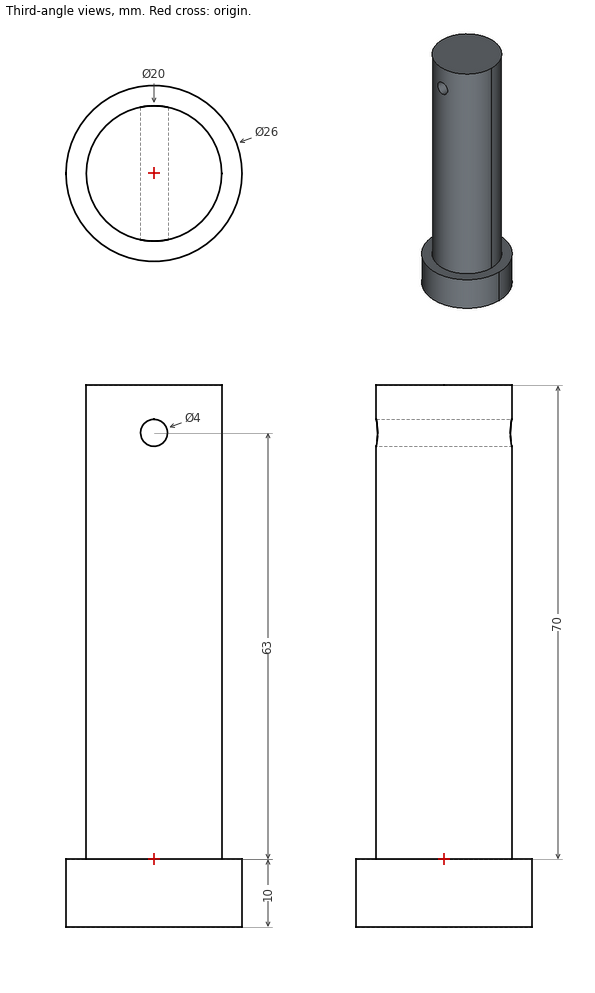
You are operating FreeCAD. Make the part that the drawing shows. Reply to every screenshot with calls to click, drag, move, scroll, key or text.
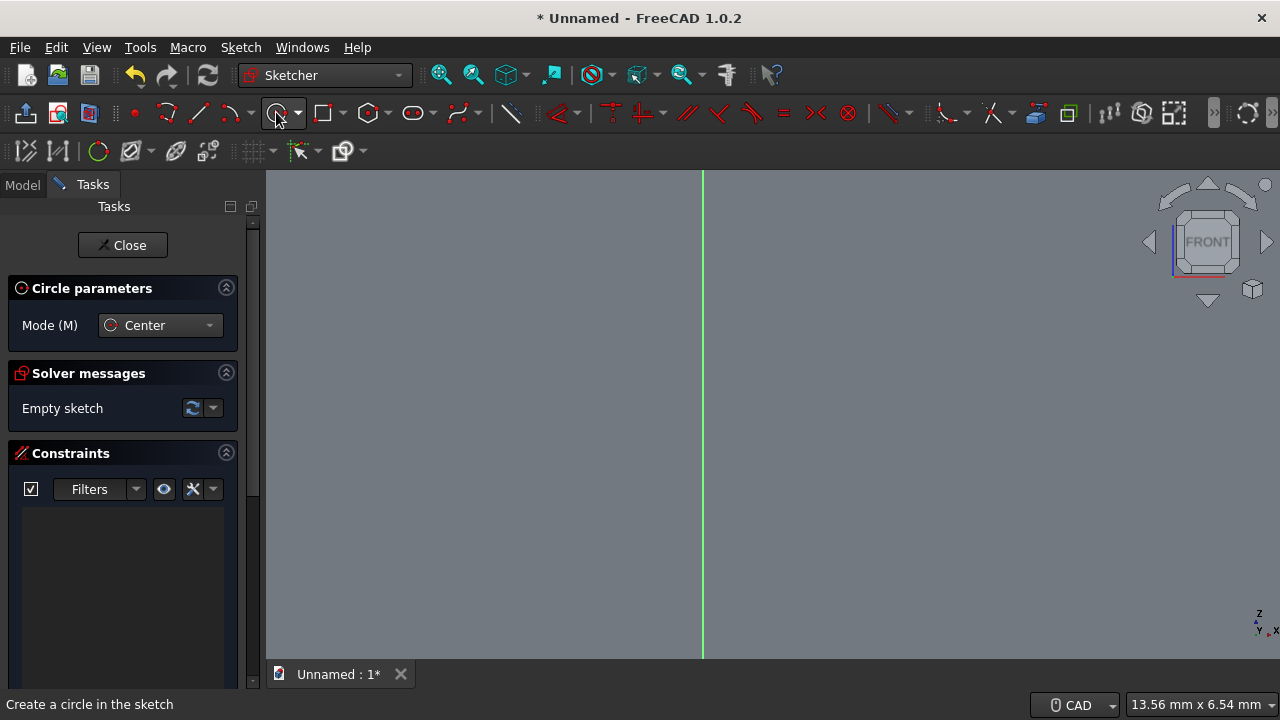
click(703, 409)
move(809, 303)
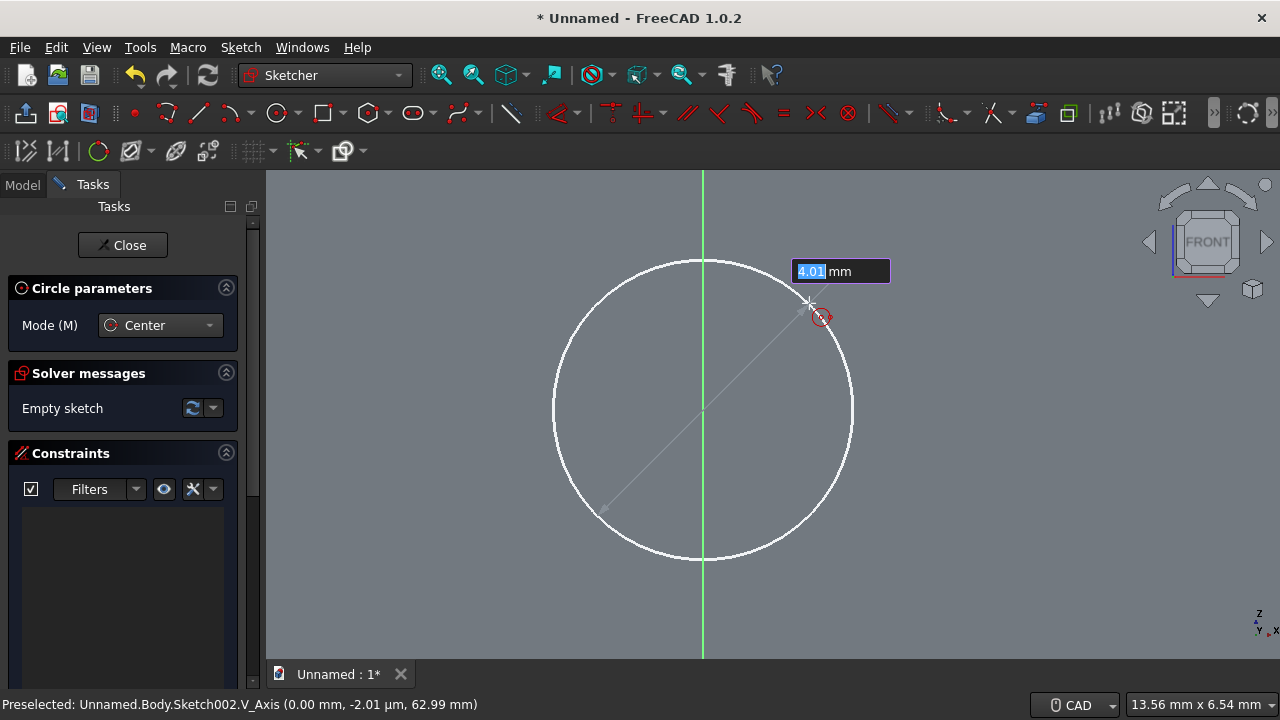
text(4)
key(Return)
key(Escape)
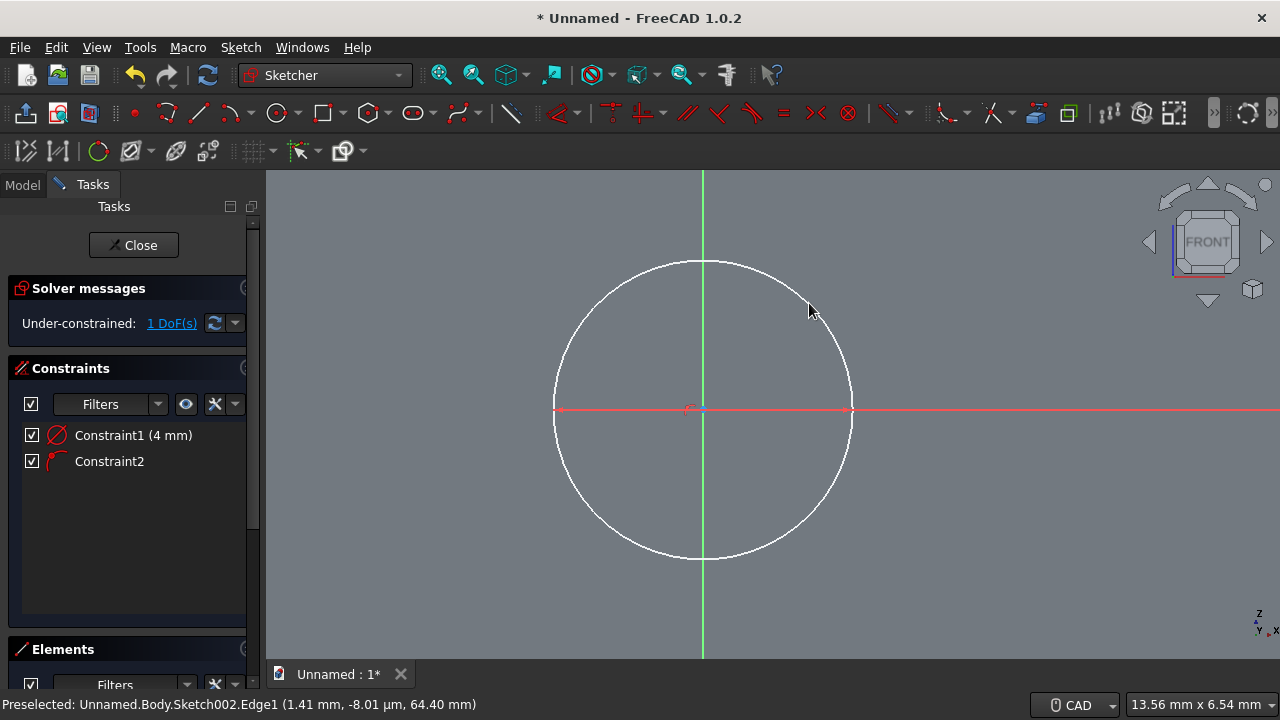
click(703, 410)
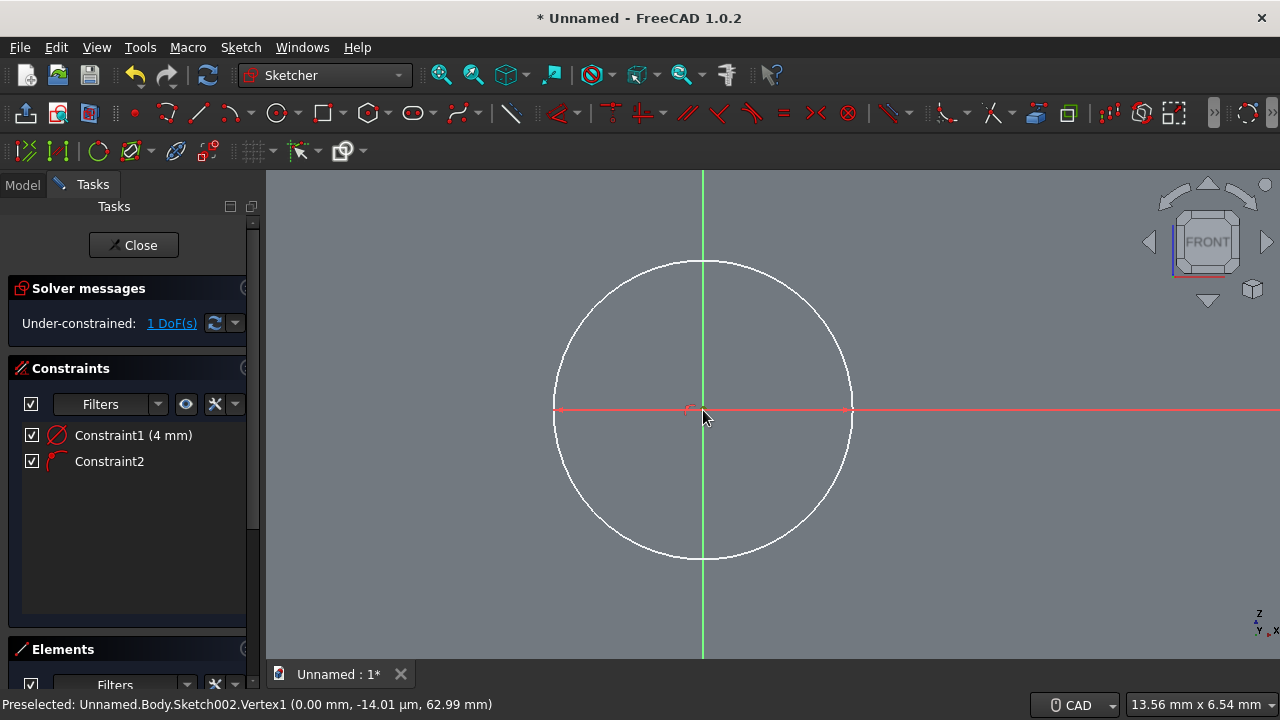
key(i)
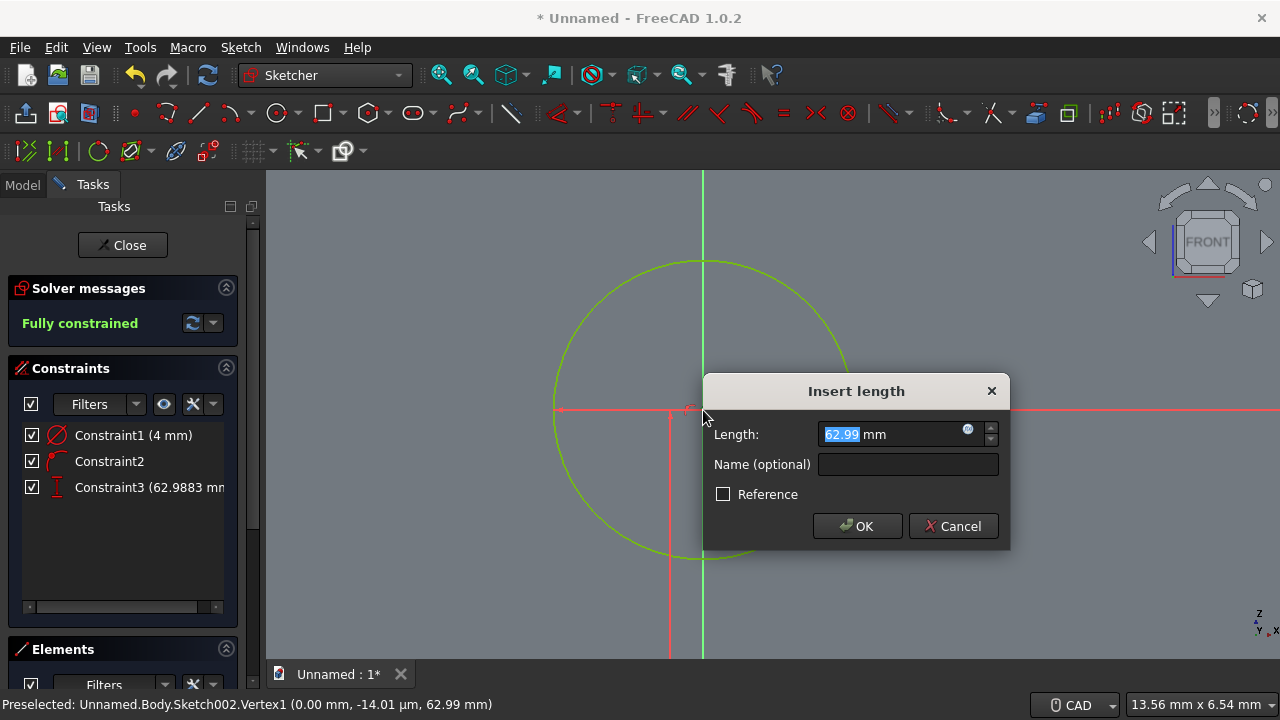
text(63)
key(Return)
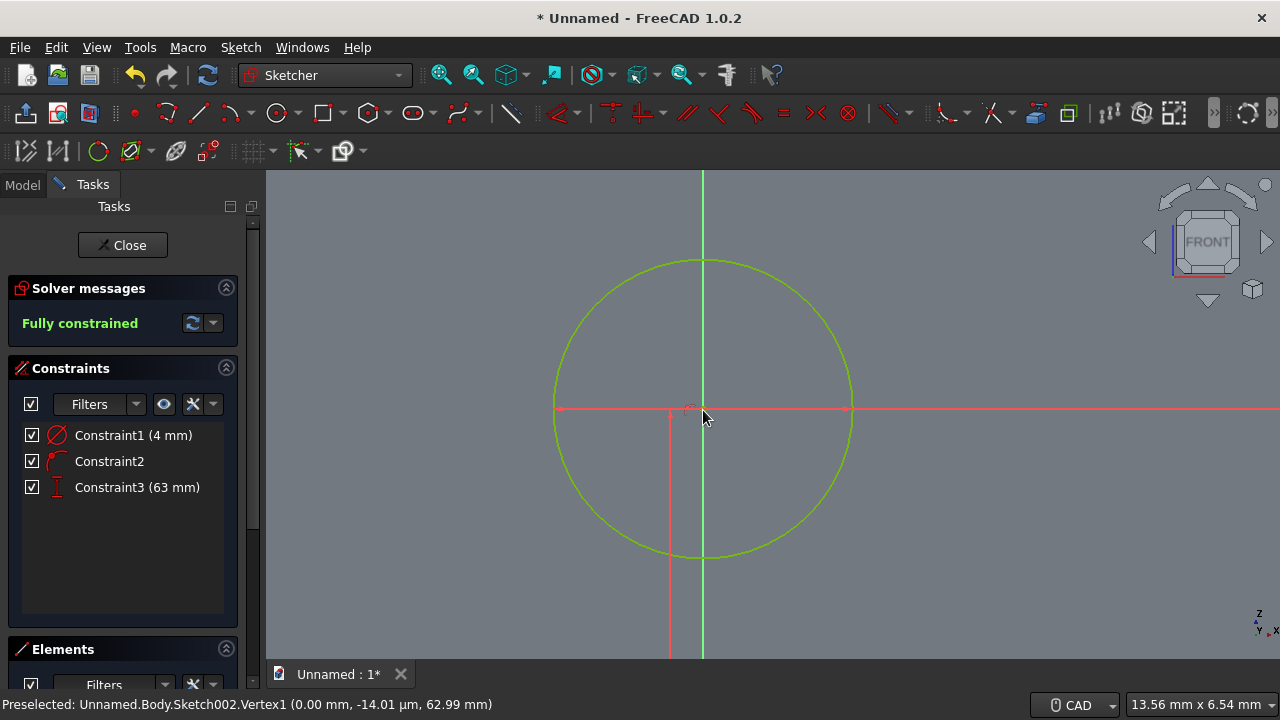
click(123, 245)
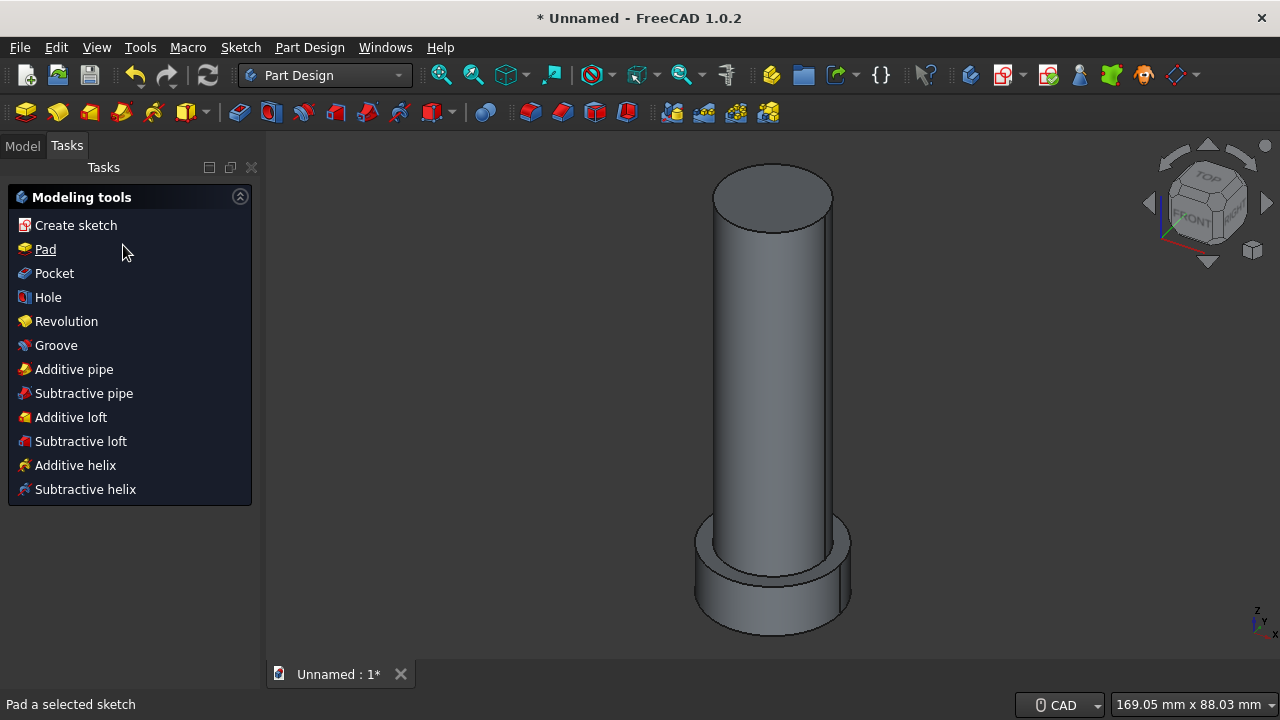
click(240, 112)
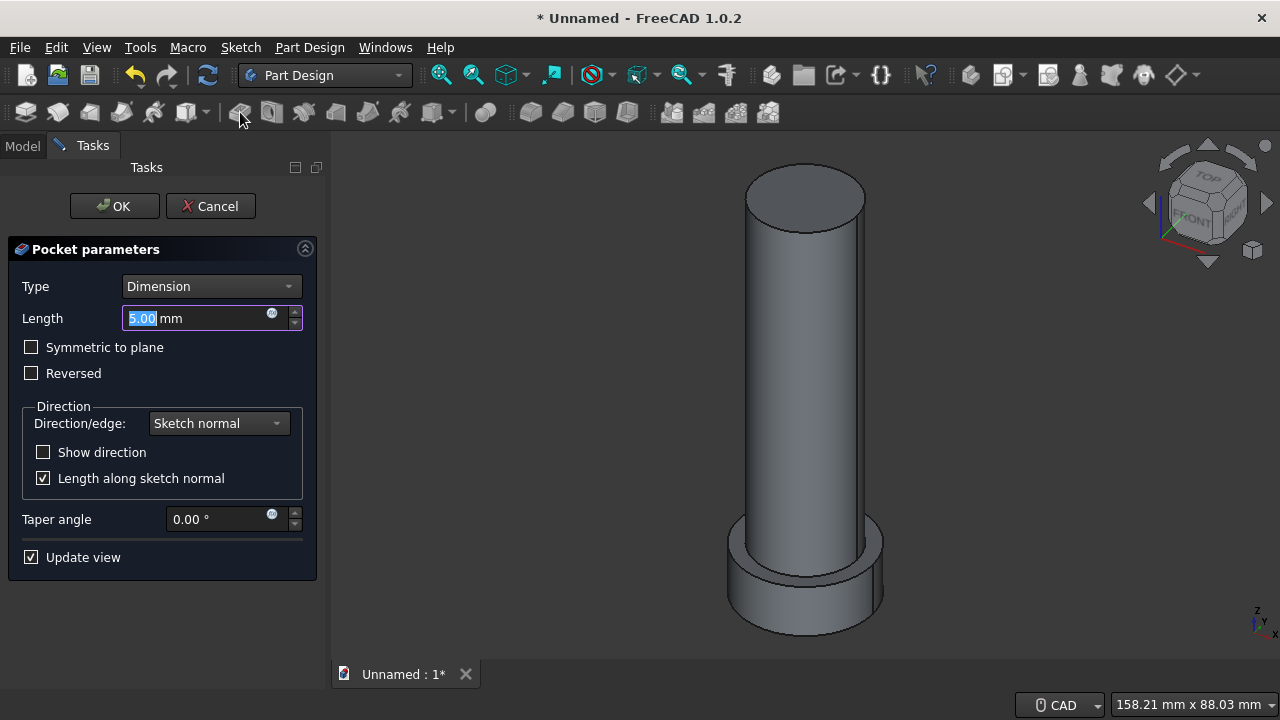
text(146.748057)
key(Tab)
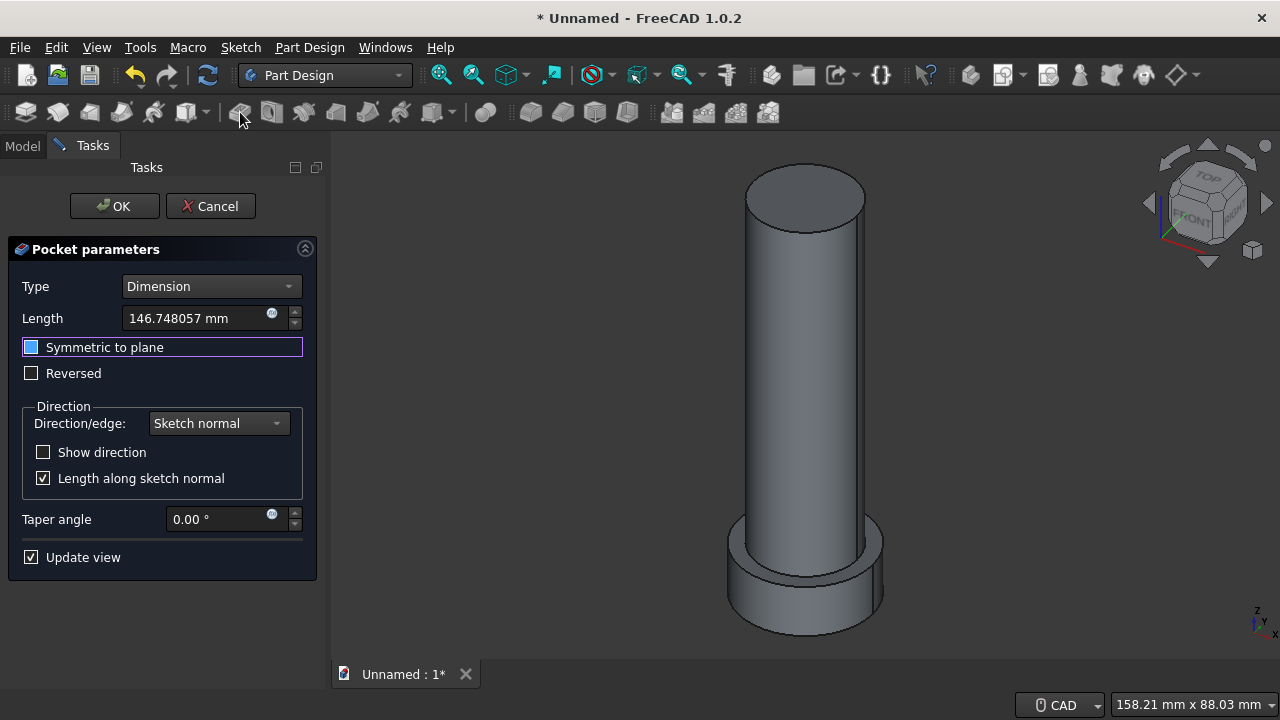
click(30, 347)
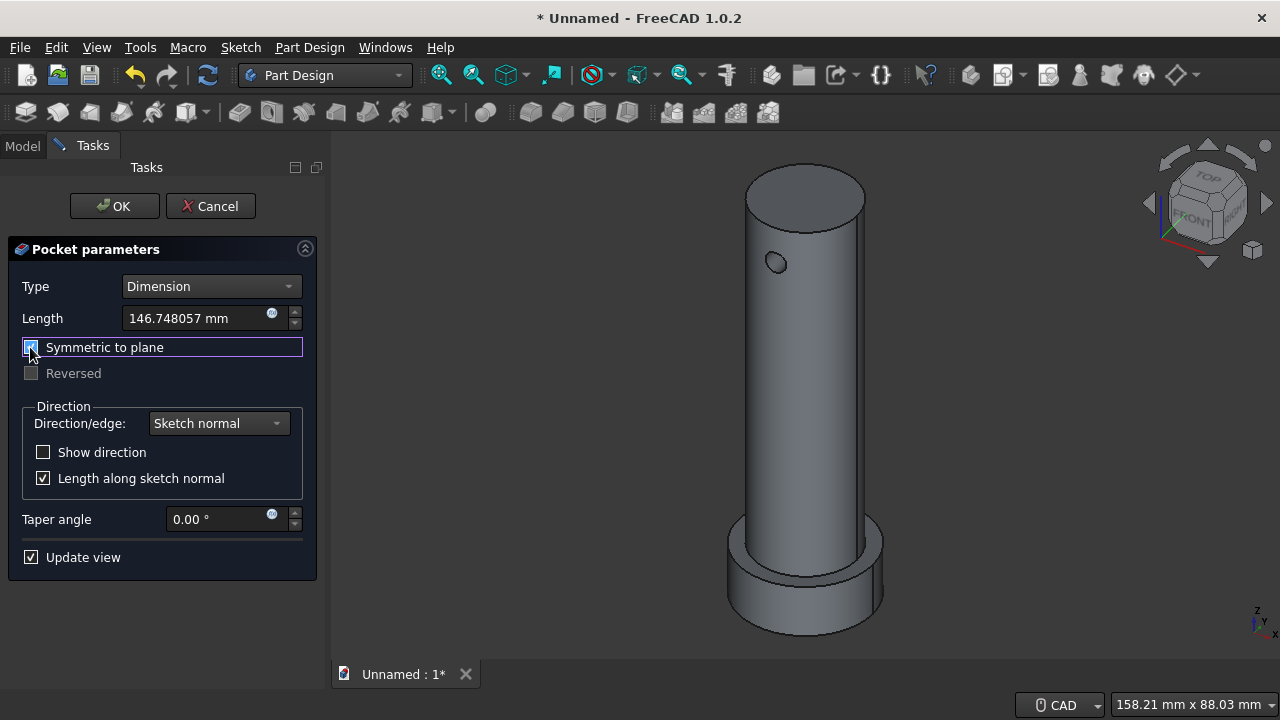
click(115, 206)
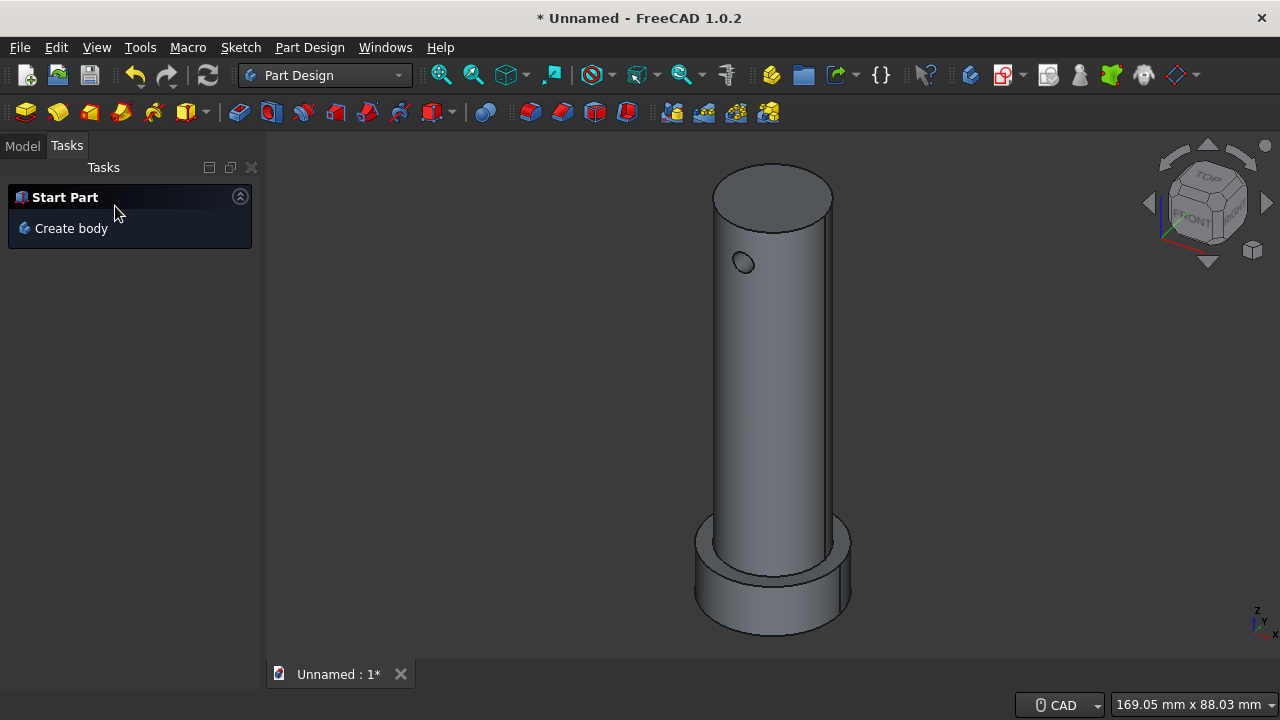
key(0)